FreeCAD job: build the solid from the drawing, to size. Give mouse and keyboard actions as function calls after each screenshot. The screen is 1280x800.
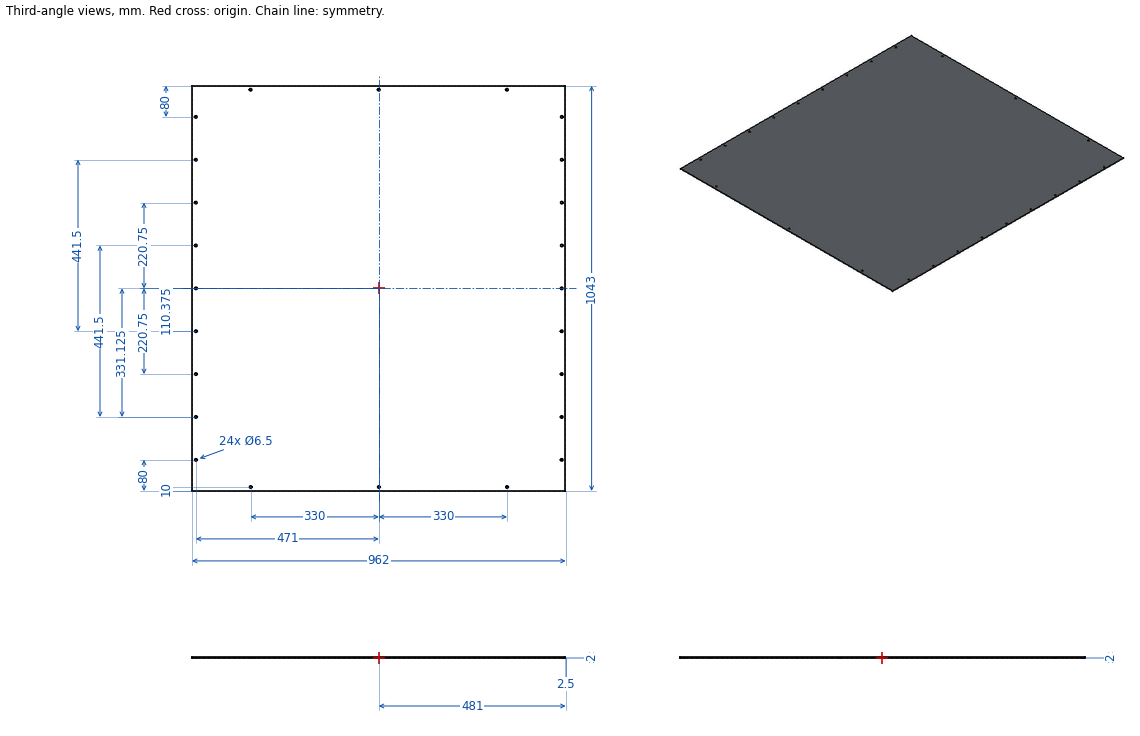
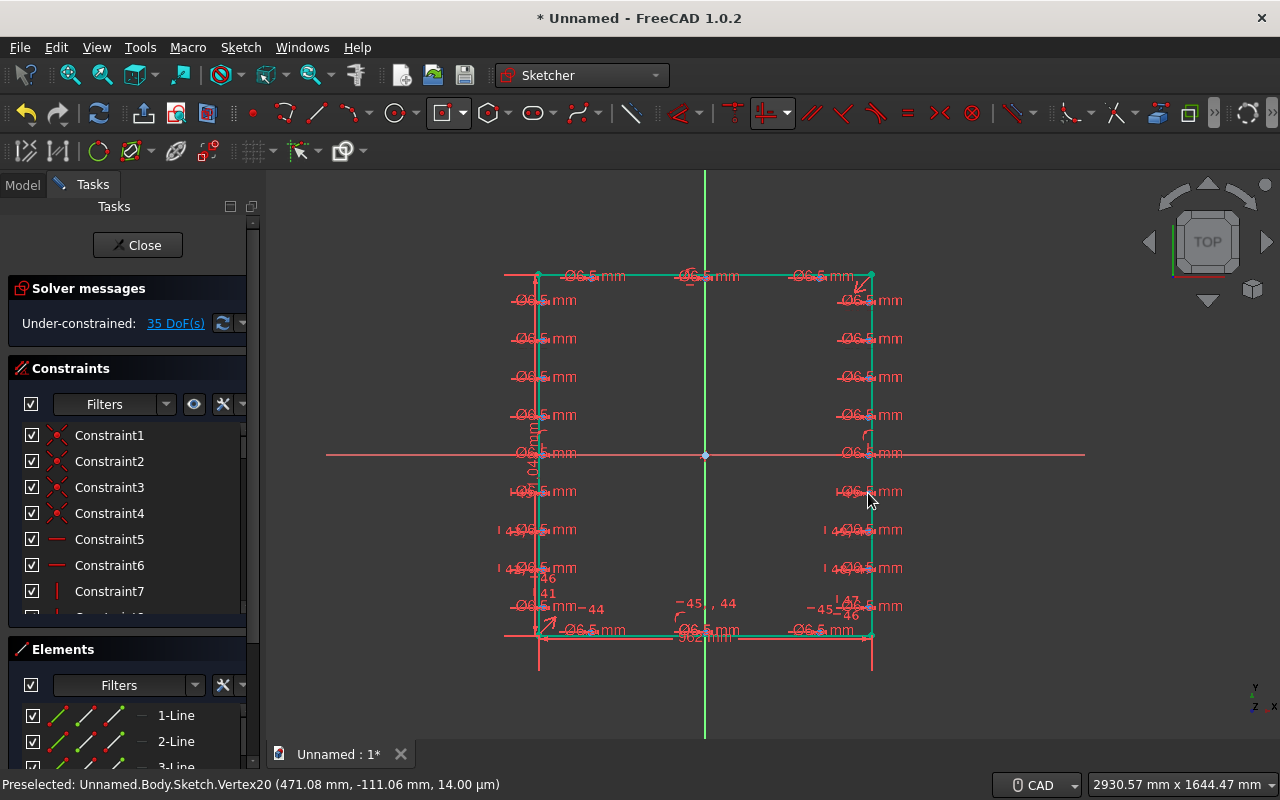
click(542, 493)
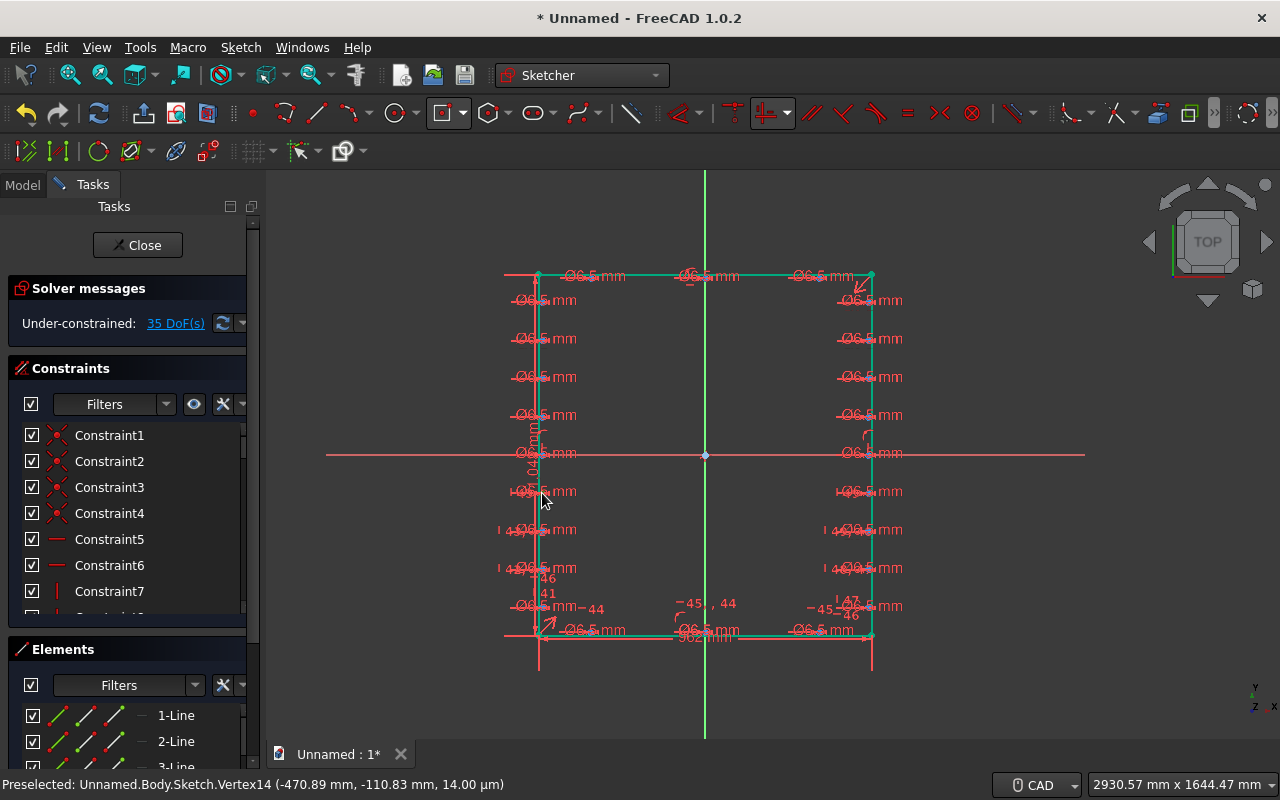
click(542, 455)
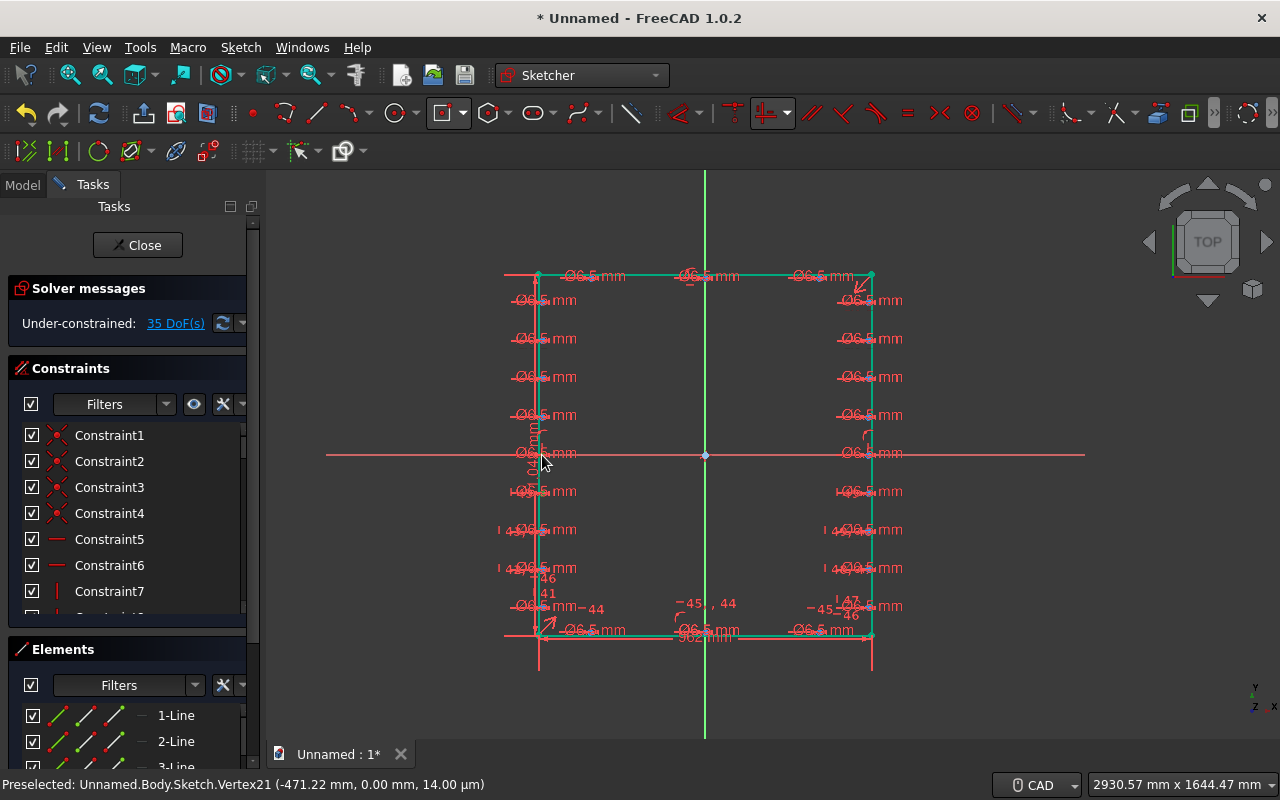
key(v)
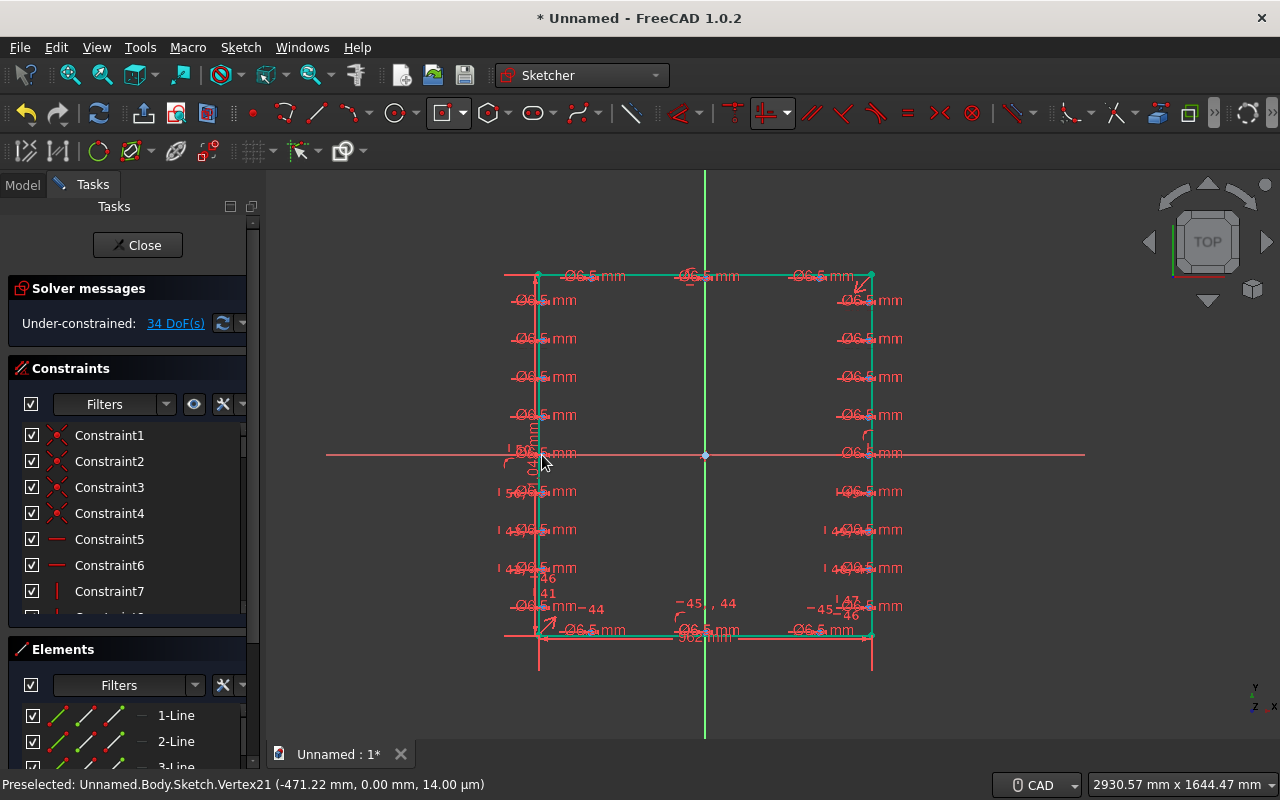
click(542, 455)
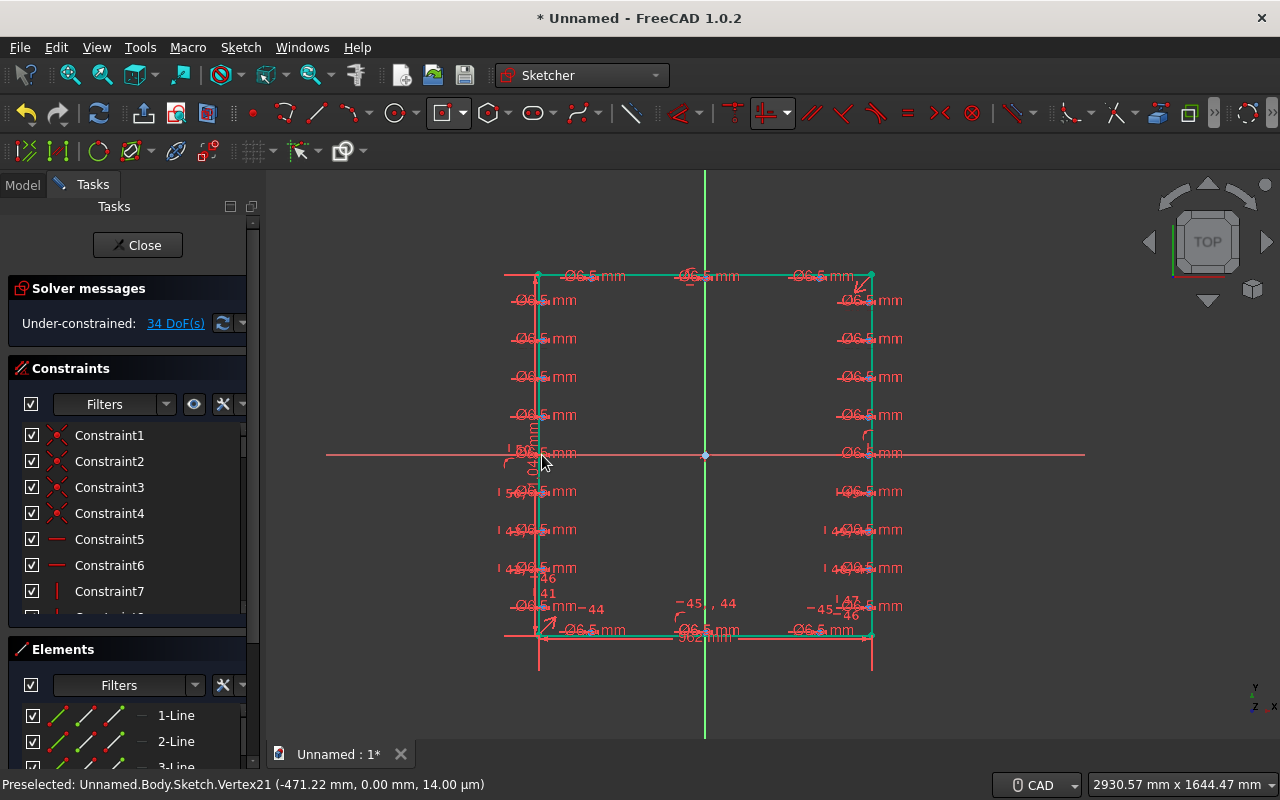
click(542, 417)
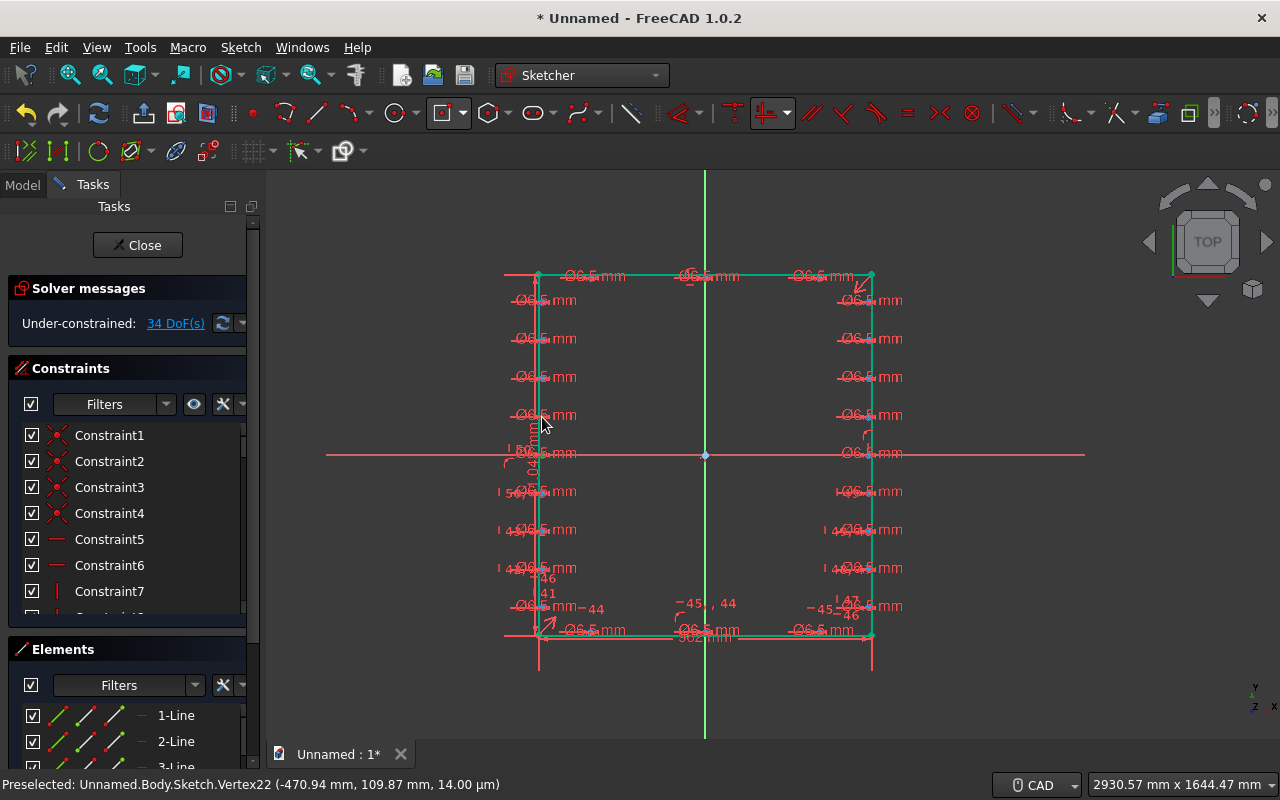
key(v)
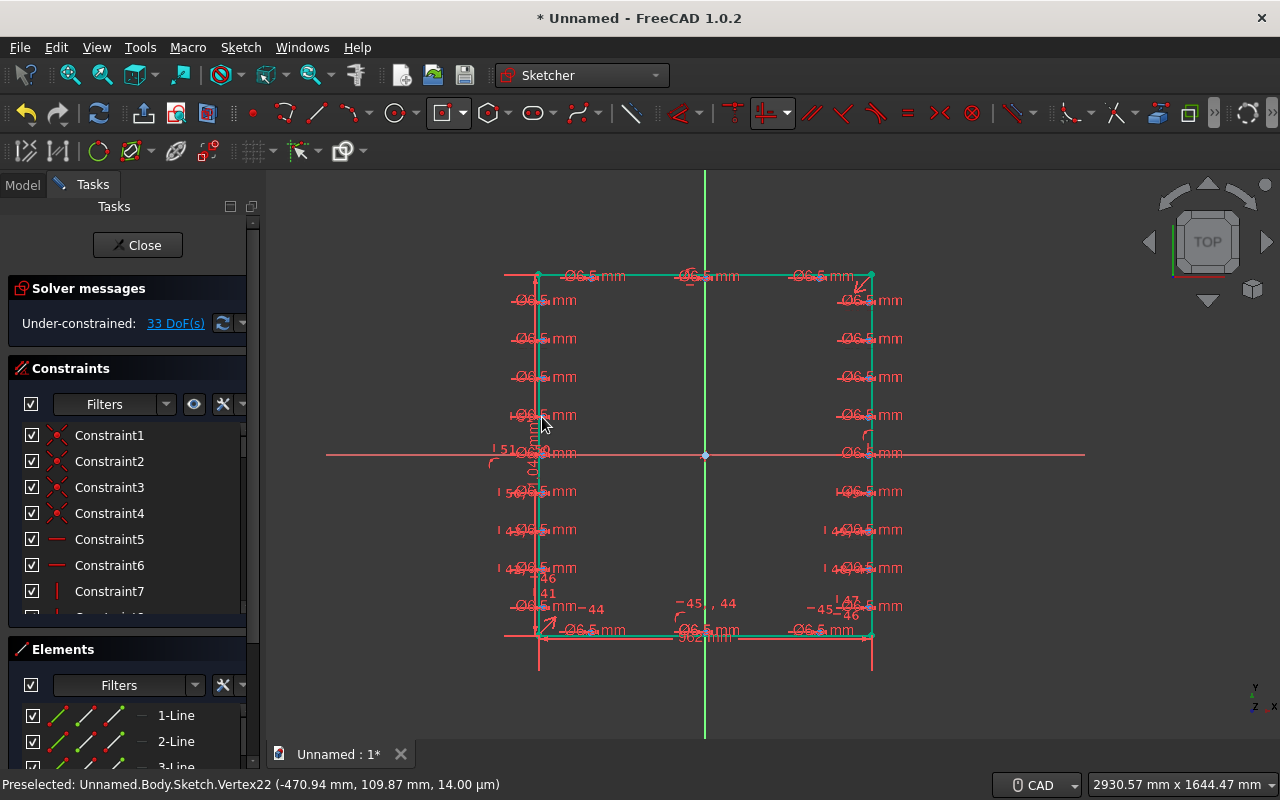
click(542, 417)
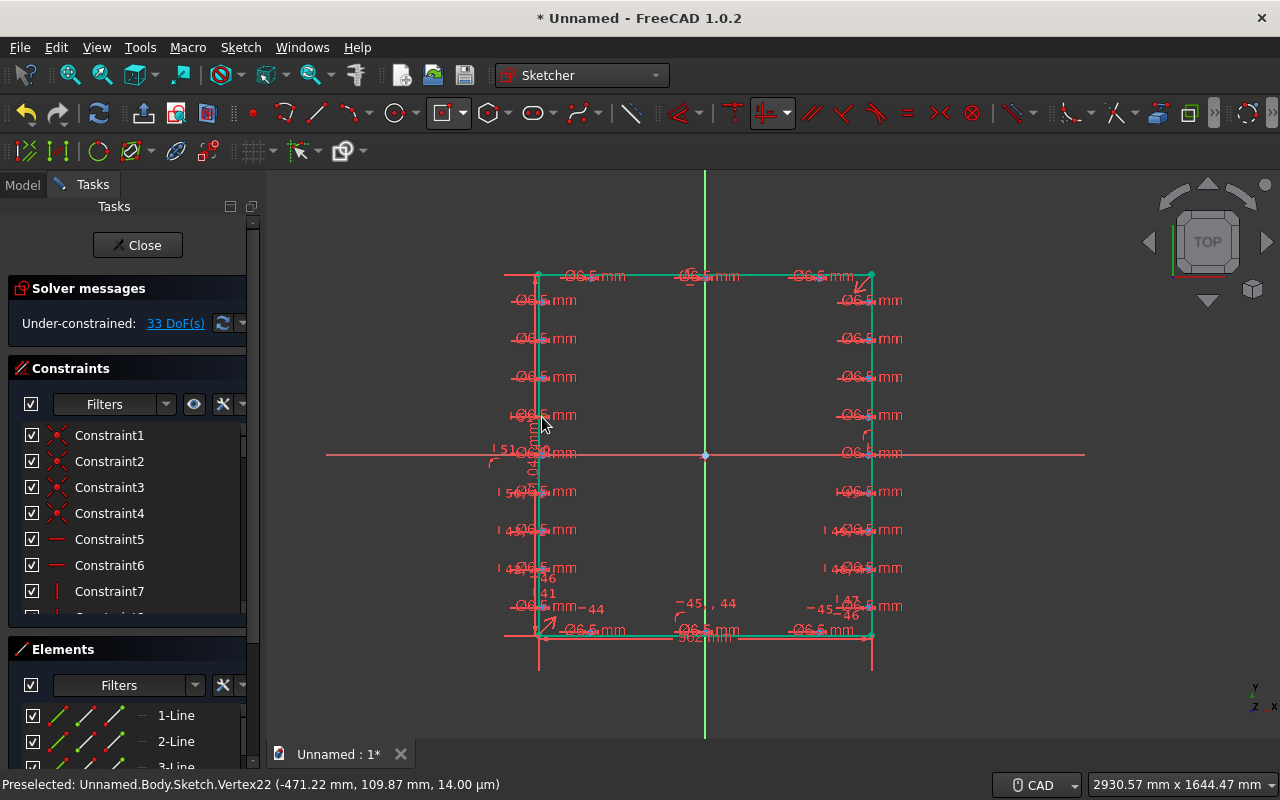
click(542, 379)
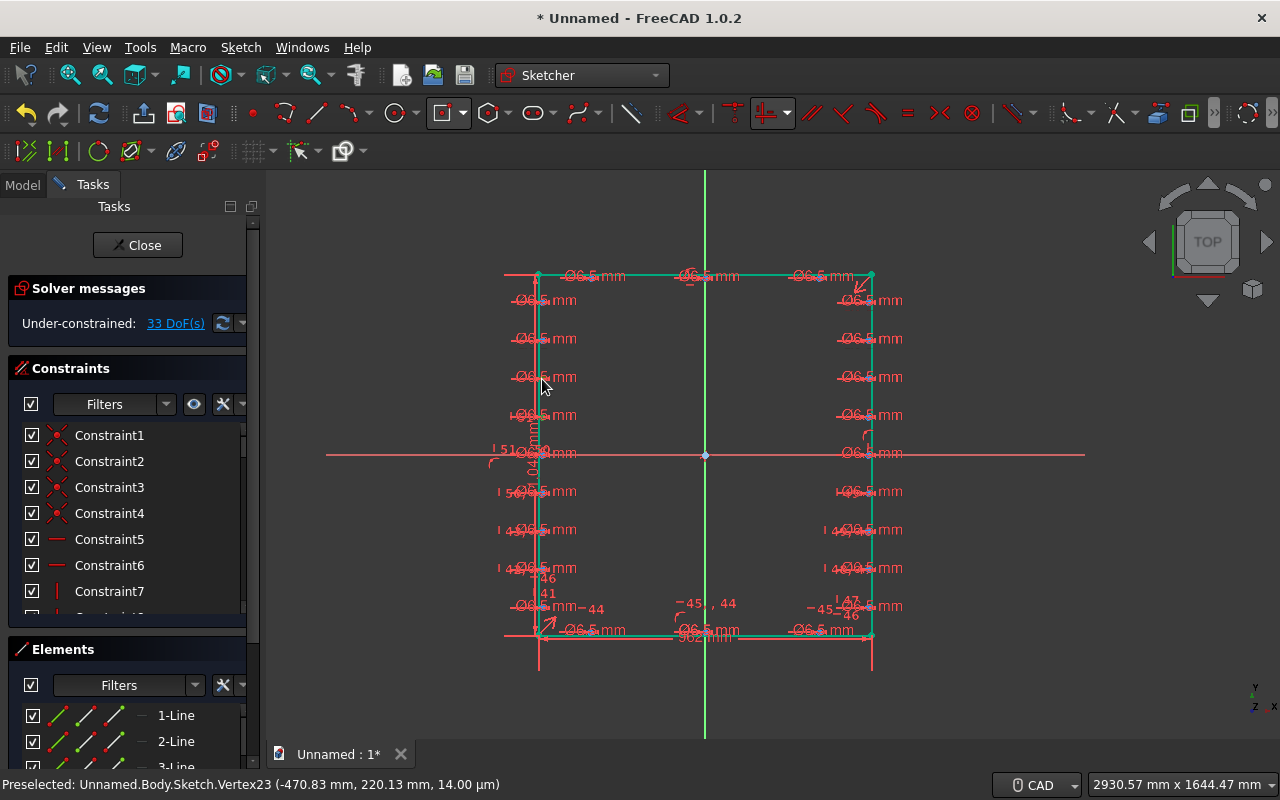
key(v)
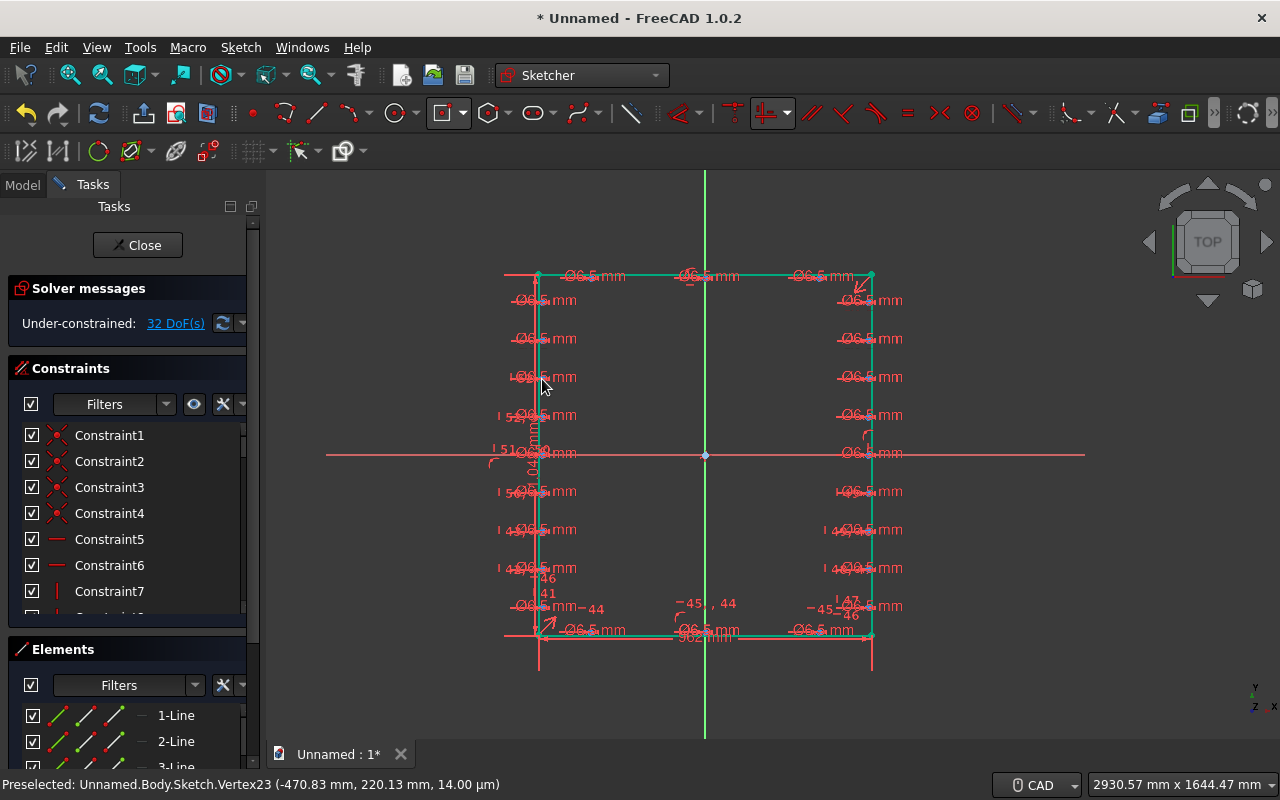
click(542, 379)